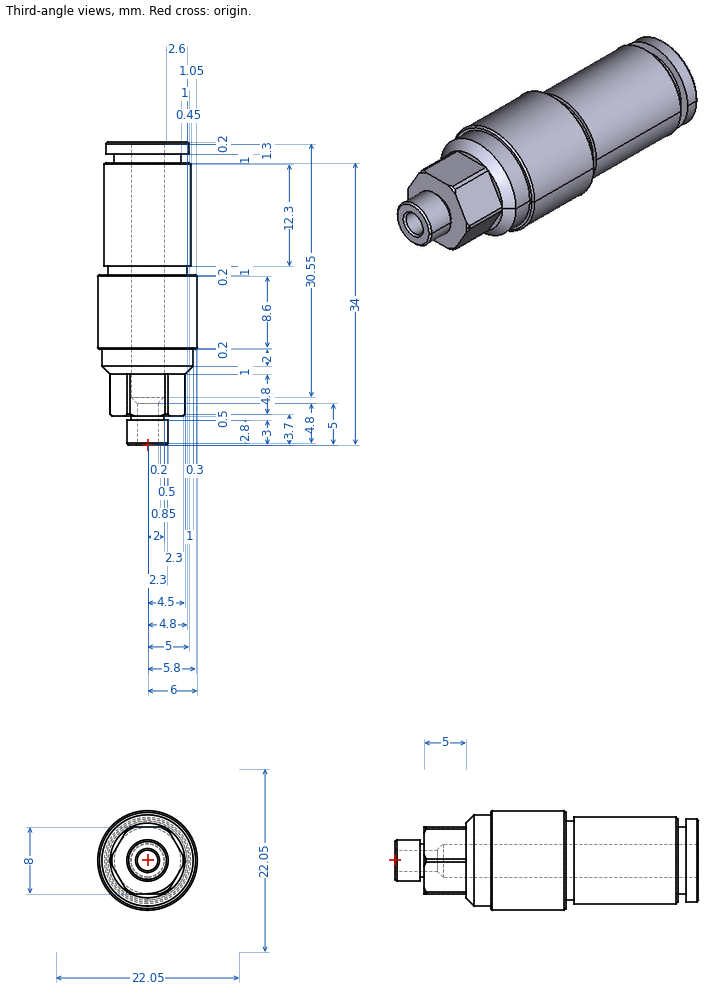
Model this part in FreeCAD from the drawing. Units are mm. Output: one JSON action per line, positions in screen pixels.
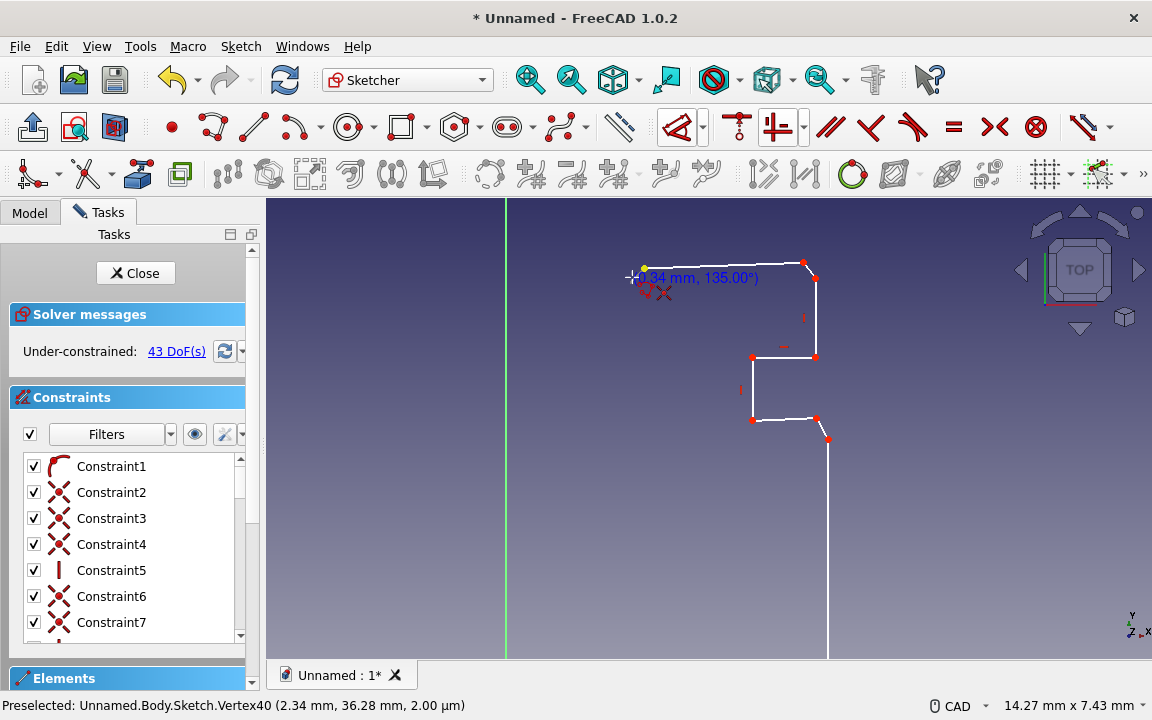
{"action": "left_click", "coordinate": [630, 275]}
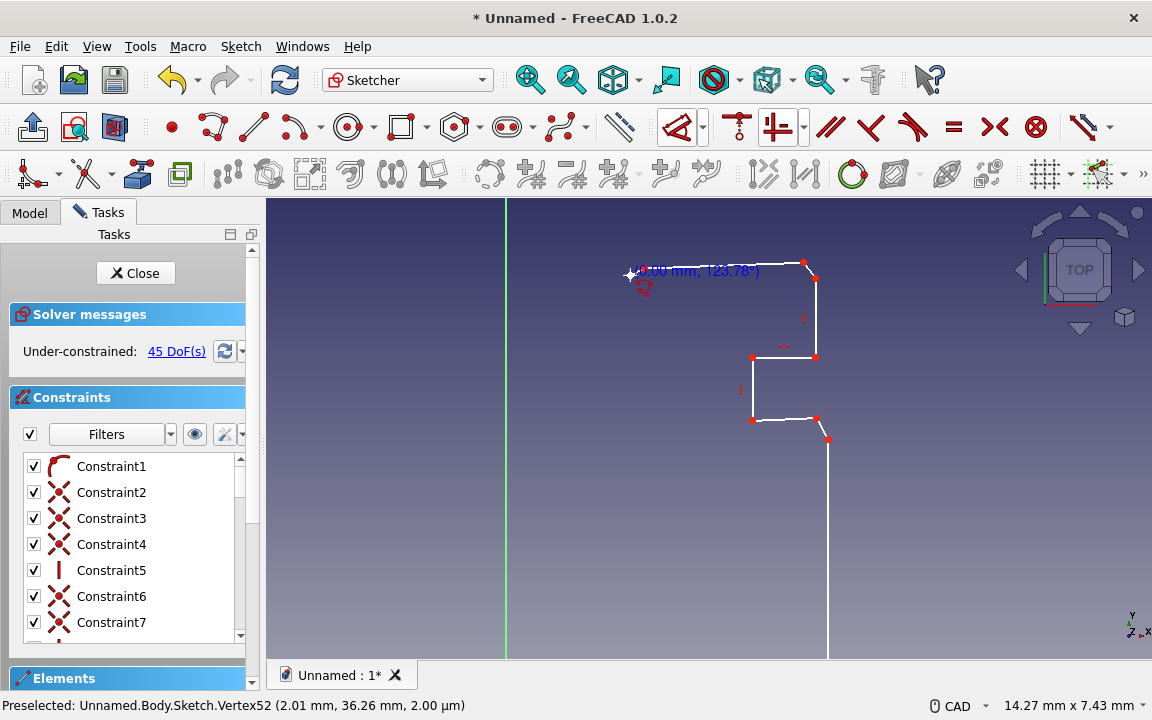
{"action": "scroll", "coordinate": [632, 277], "scroll_direction": "down", "scroll_amount": 10}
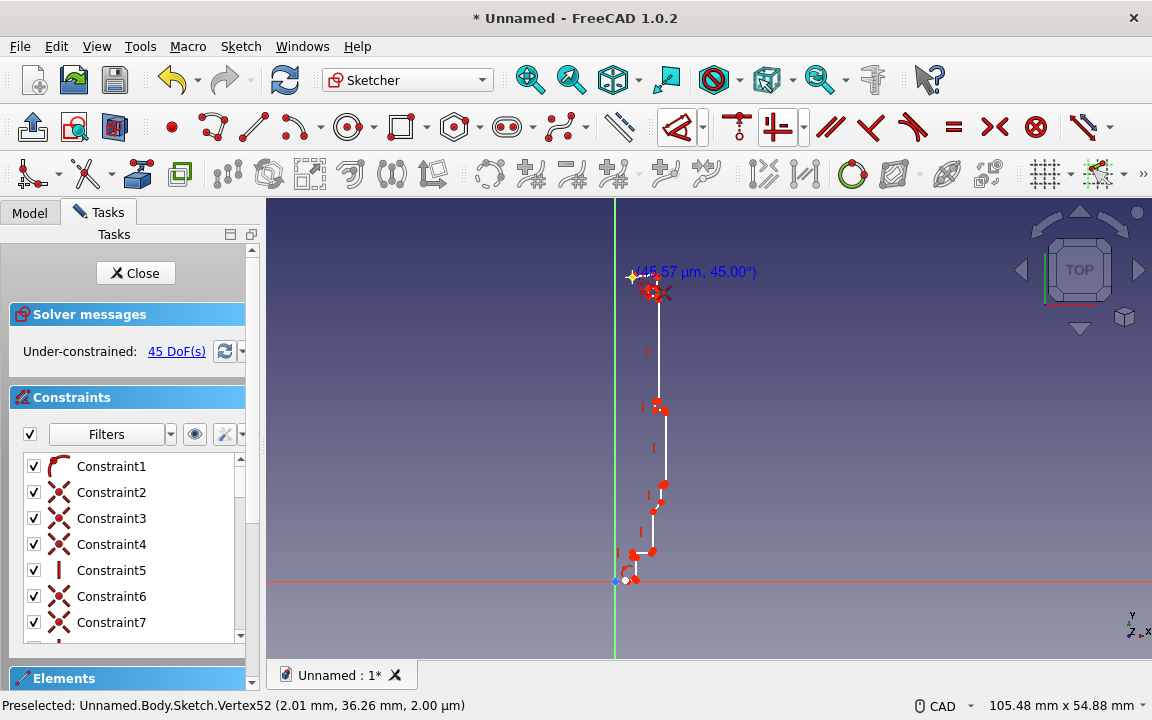
{"action": "left_click", "coordinate": [632, 533]}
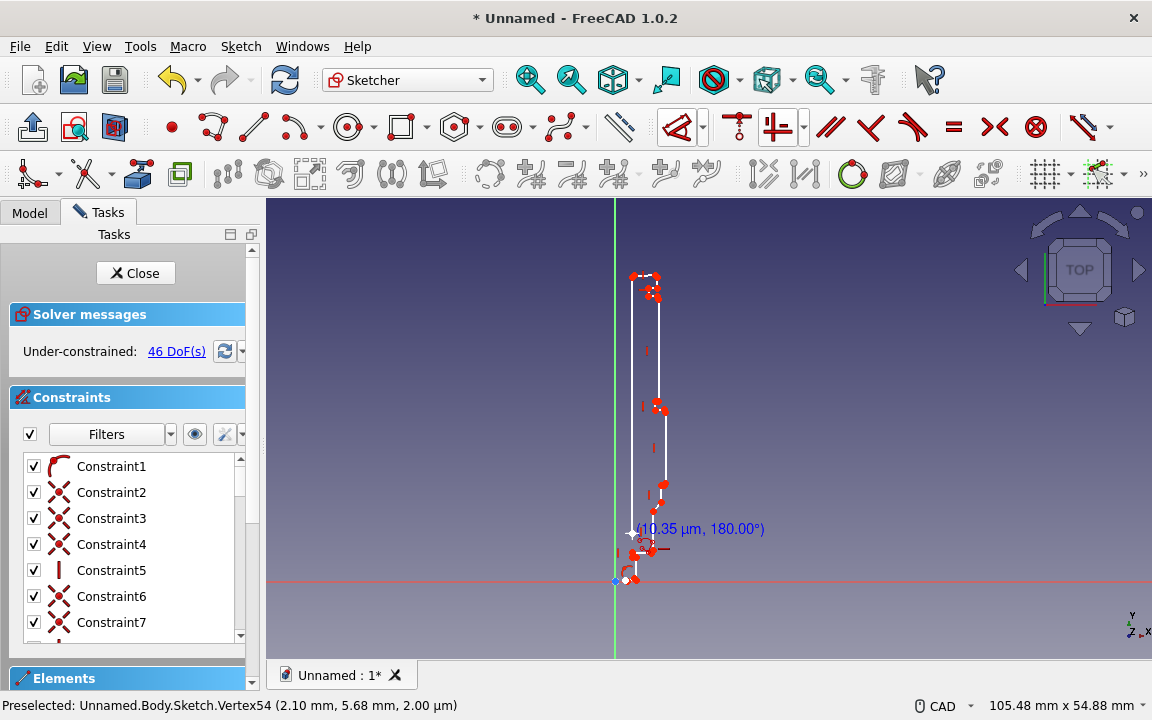
{"action": "scroll", "coordinate": [626, 540], "scroll_direction": "up", "scroll_amount": 3}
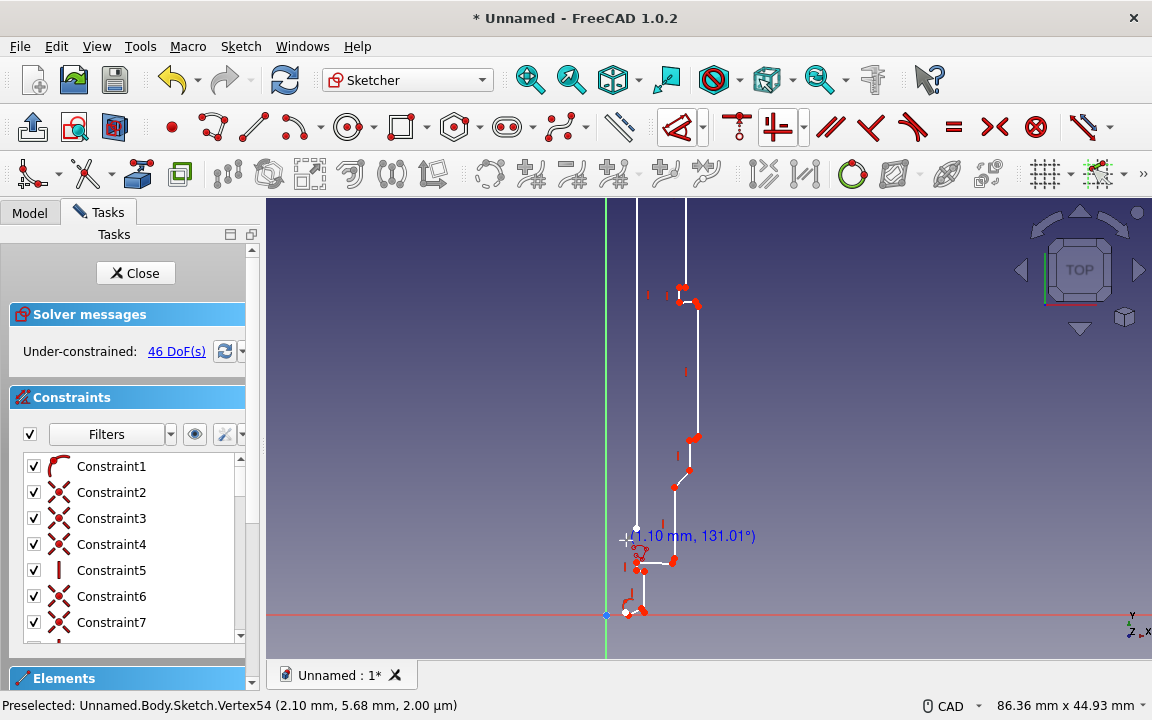
{"action": "left_click", "coordinate": [625, 539]}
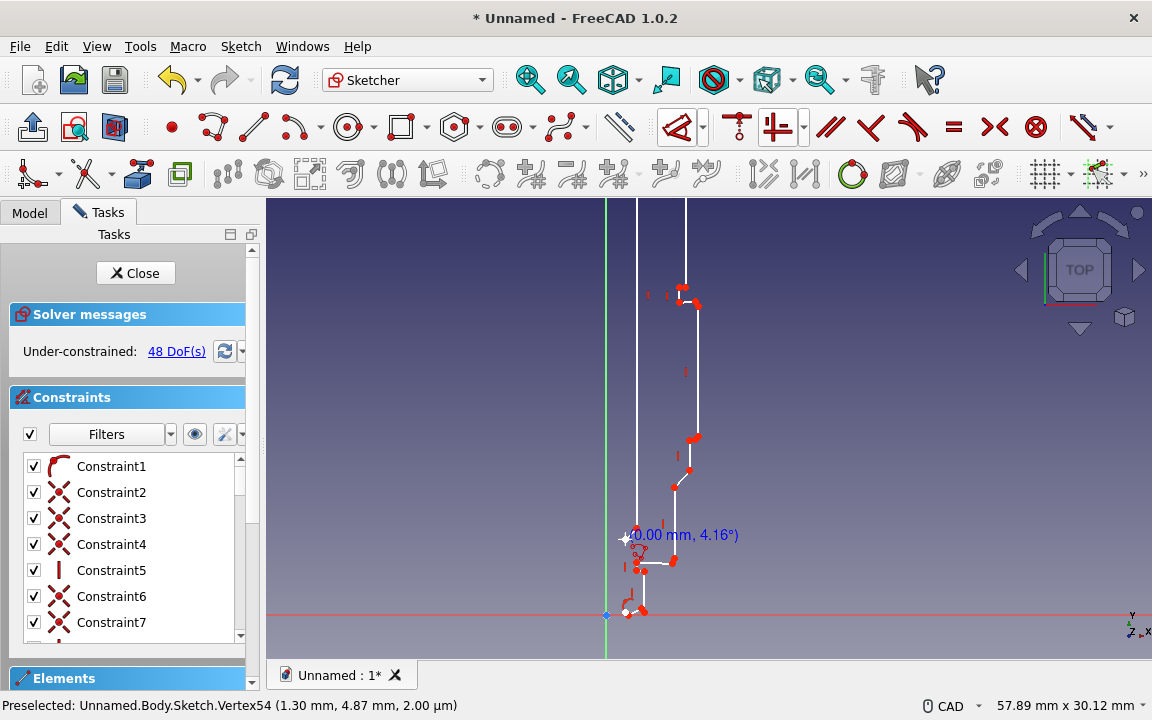
{"action": "scroll", "coordinate": [625, 612], "scroll_direction": "up", "scroll_amount": 10}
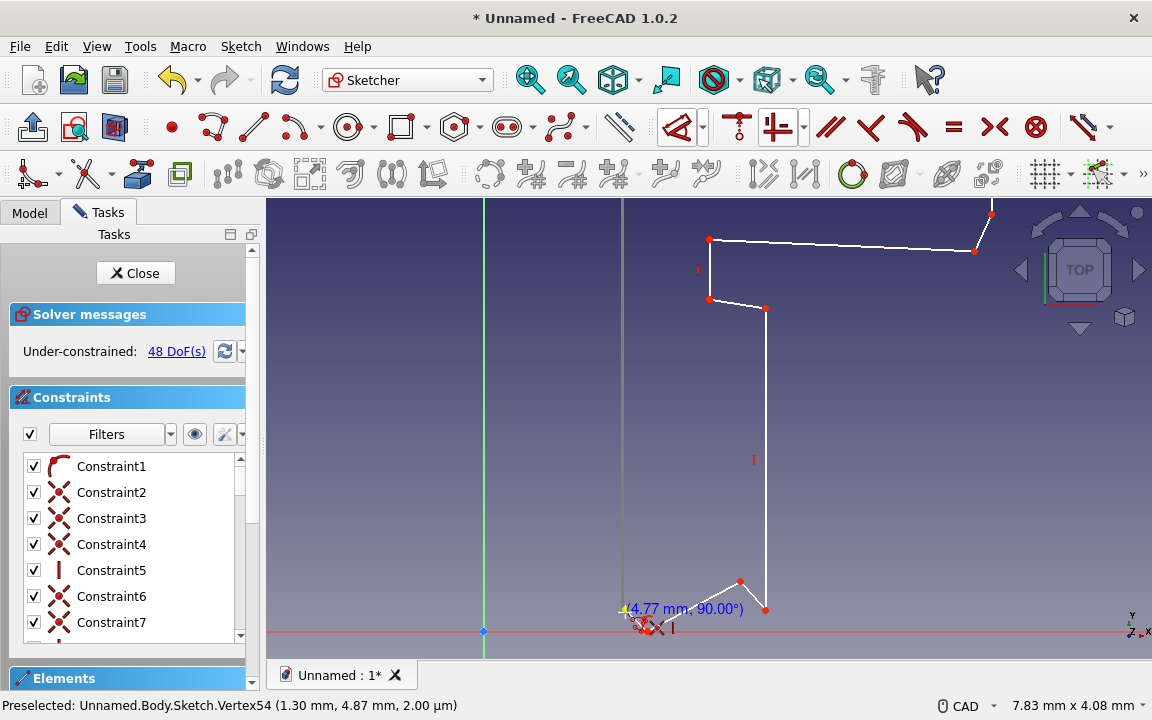
{"action": "left_click", "coordinate": [625, 610]}
{"action": "key", "text": "Escape"}
{"action": "key", "text": "Escape"}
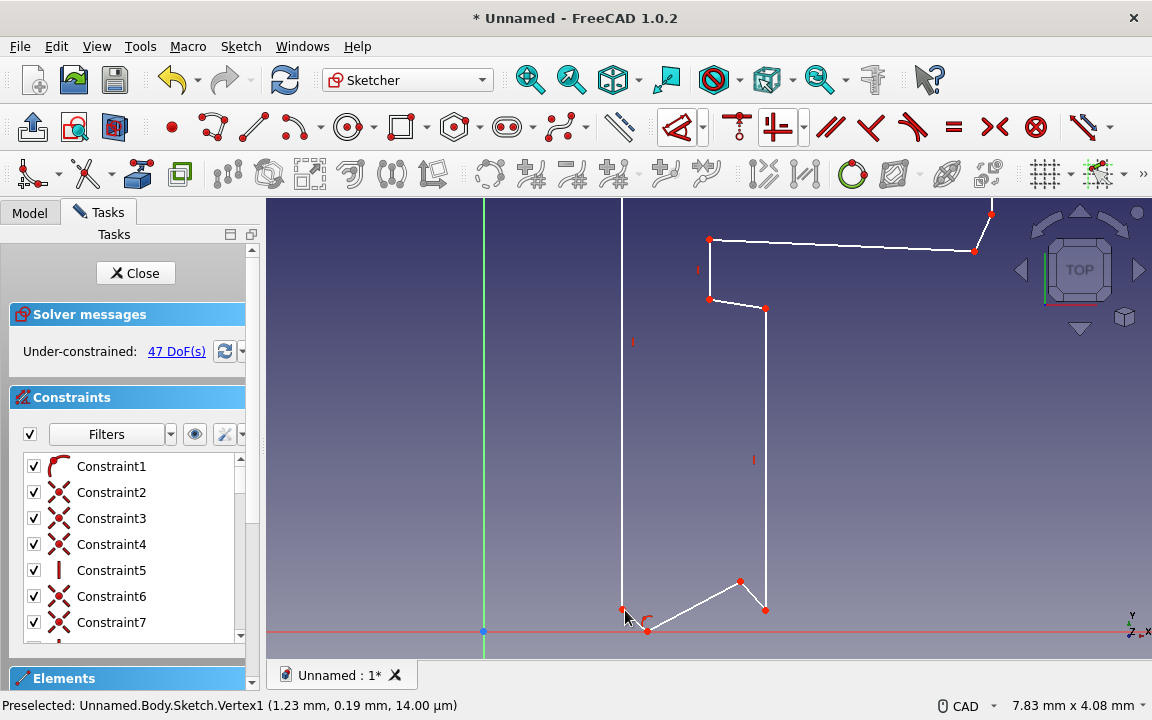
{"action": "left_click", "coordinate": [675, 617]}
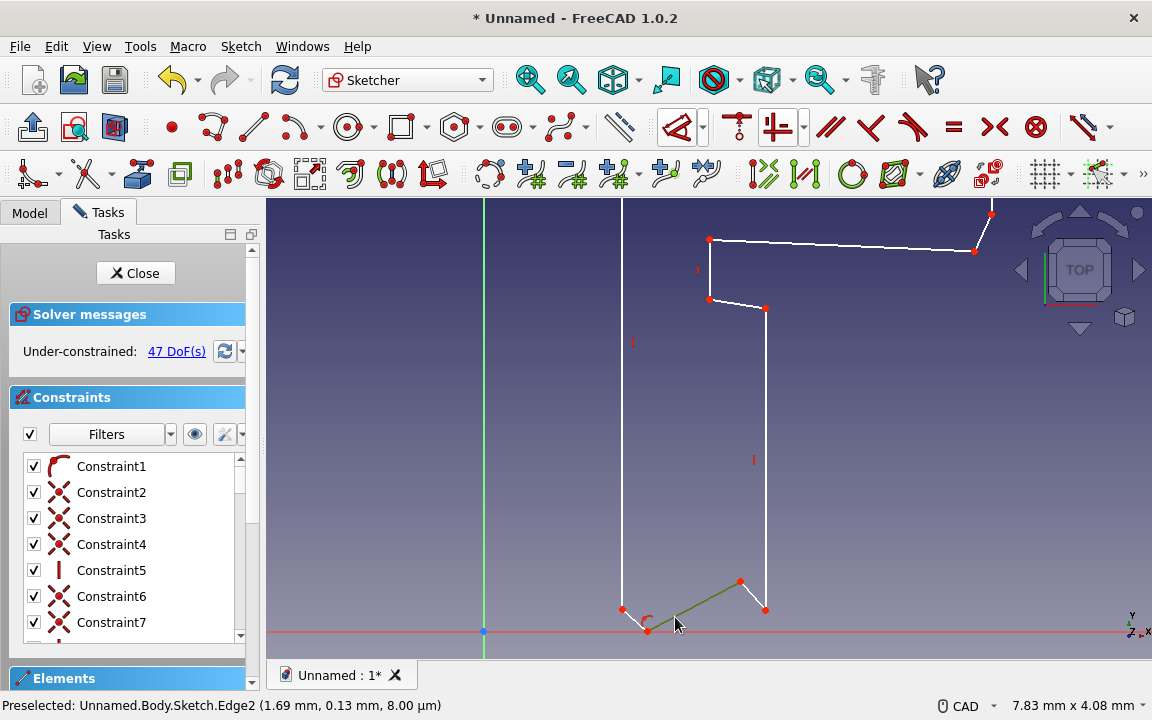
{"action": "key", "text": "h"}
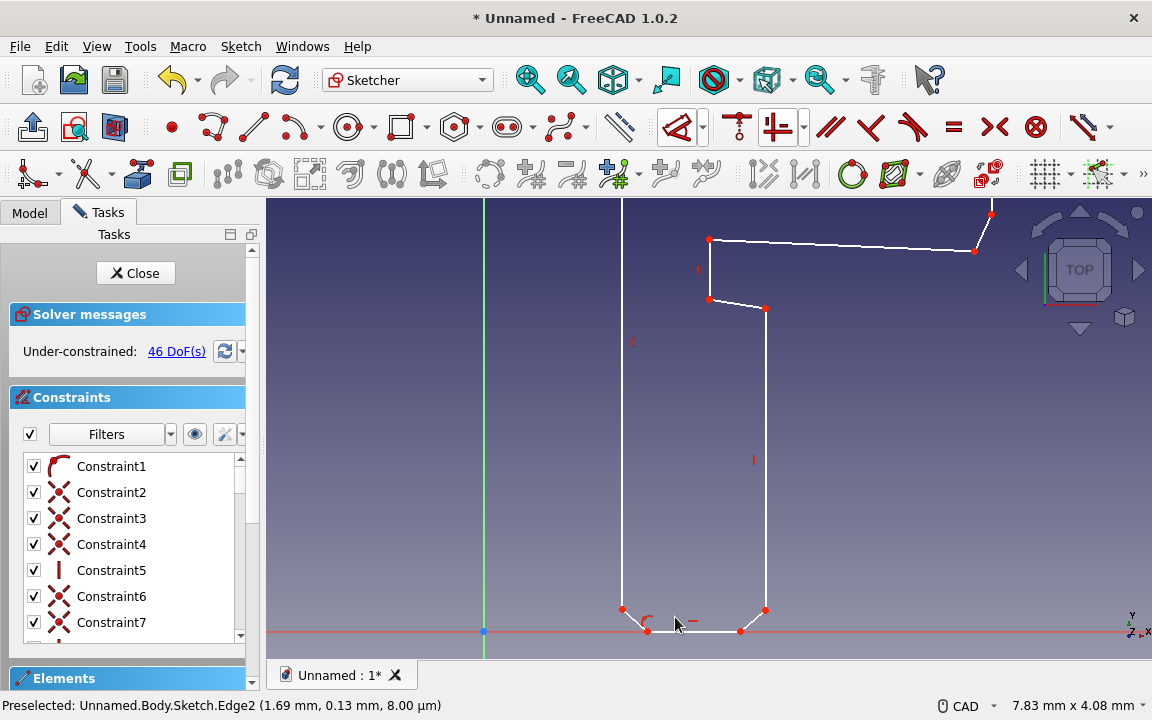
{"action": "left_click", "coordinate": [749, 306]}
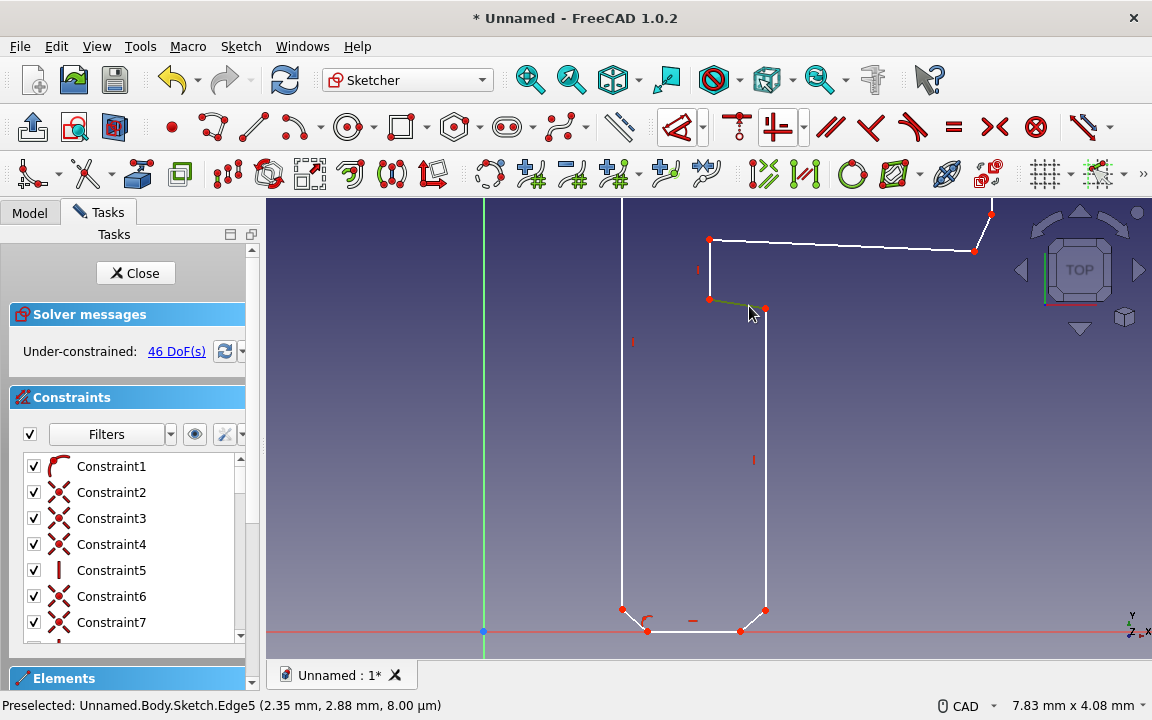
{"action": "key", "text": "h"}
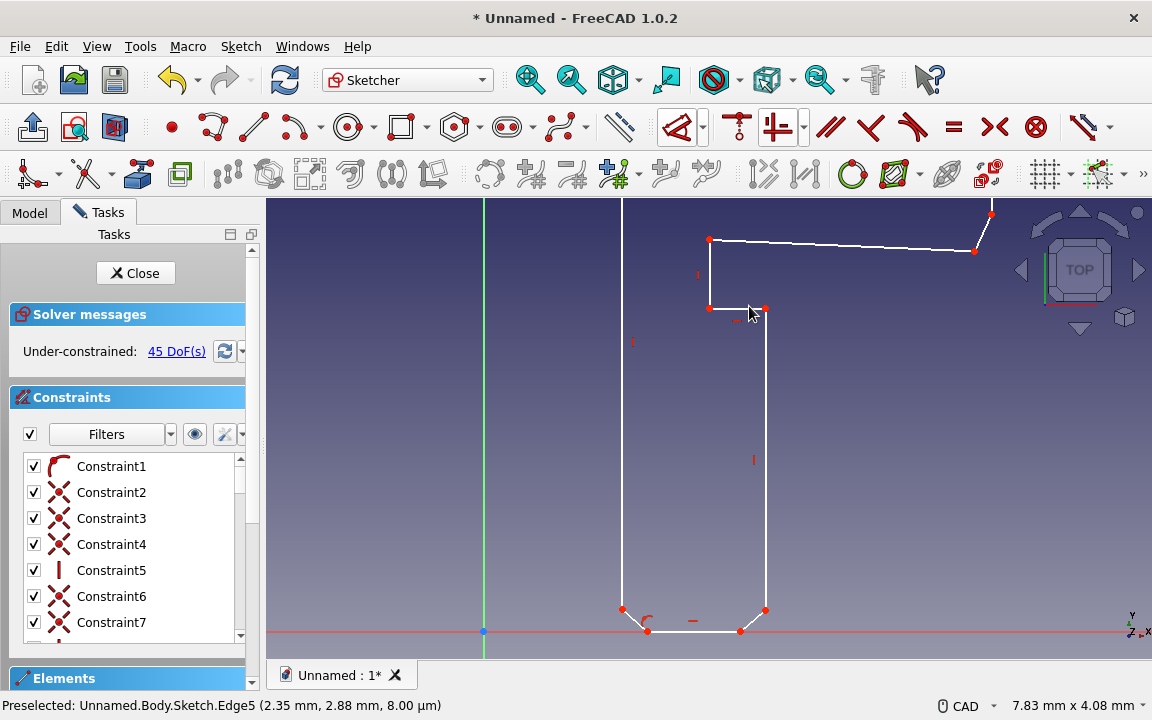
{"action": "scroll", "coordinate": [626, 578], "scroll_direction": "down", "scroll_amount": 13}